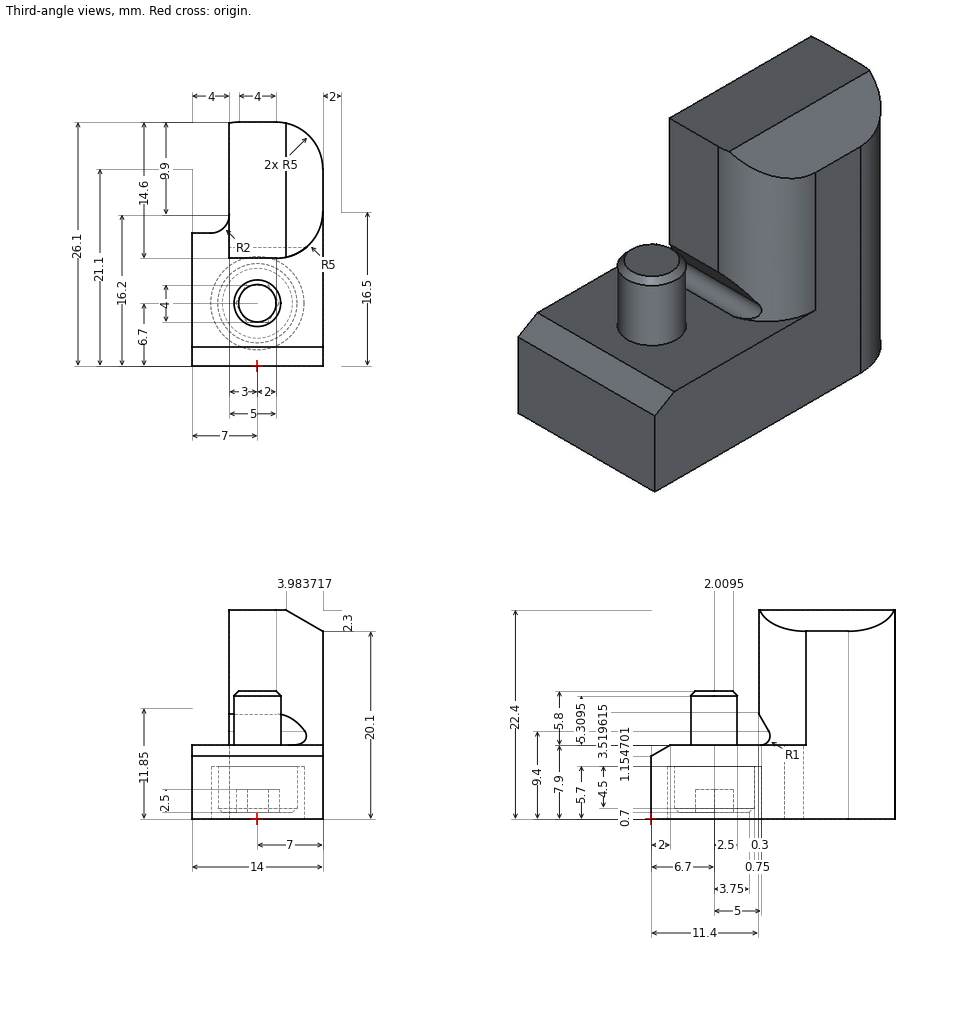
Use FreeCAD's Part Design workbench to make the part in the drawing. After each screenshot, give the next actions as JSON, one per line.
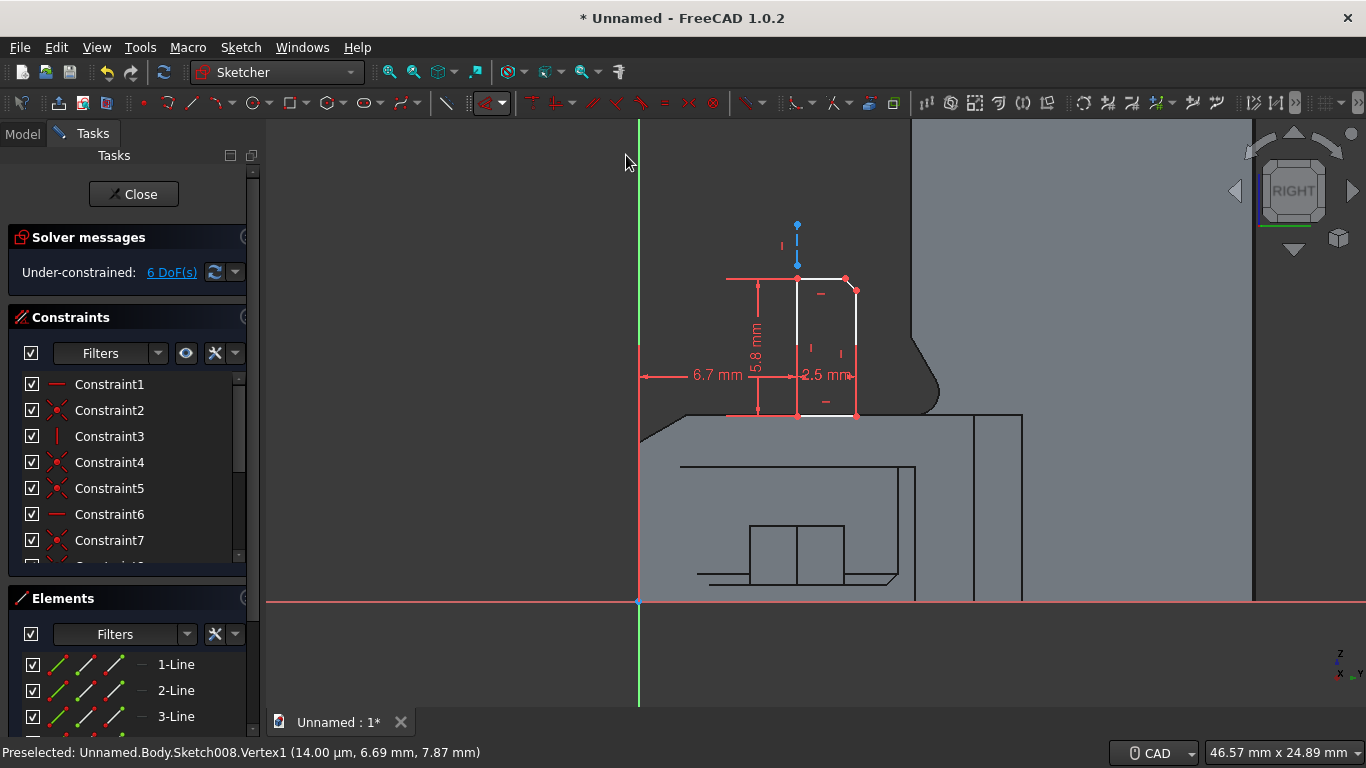
{"action": "left_click", "coordinate": [797, 416]}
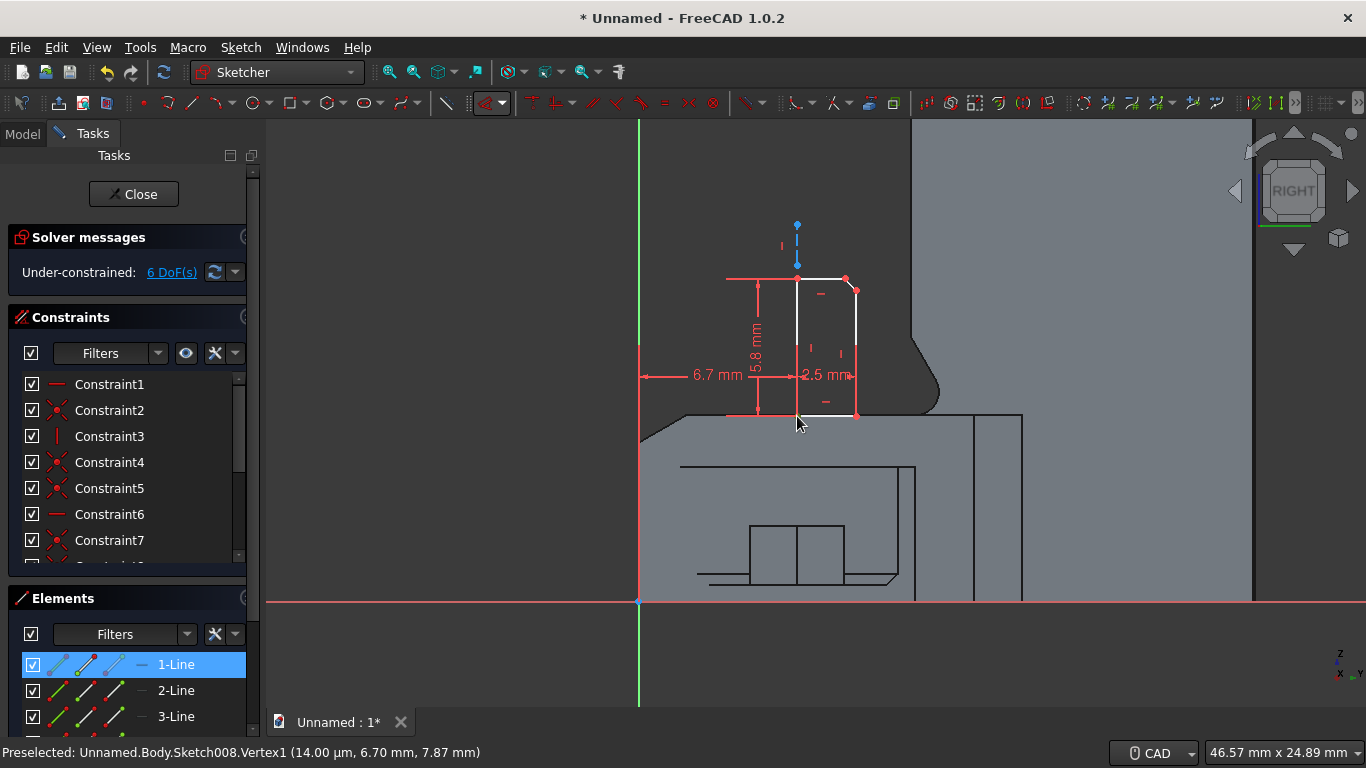
{"action": "key", "text": "i"}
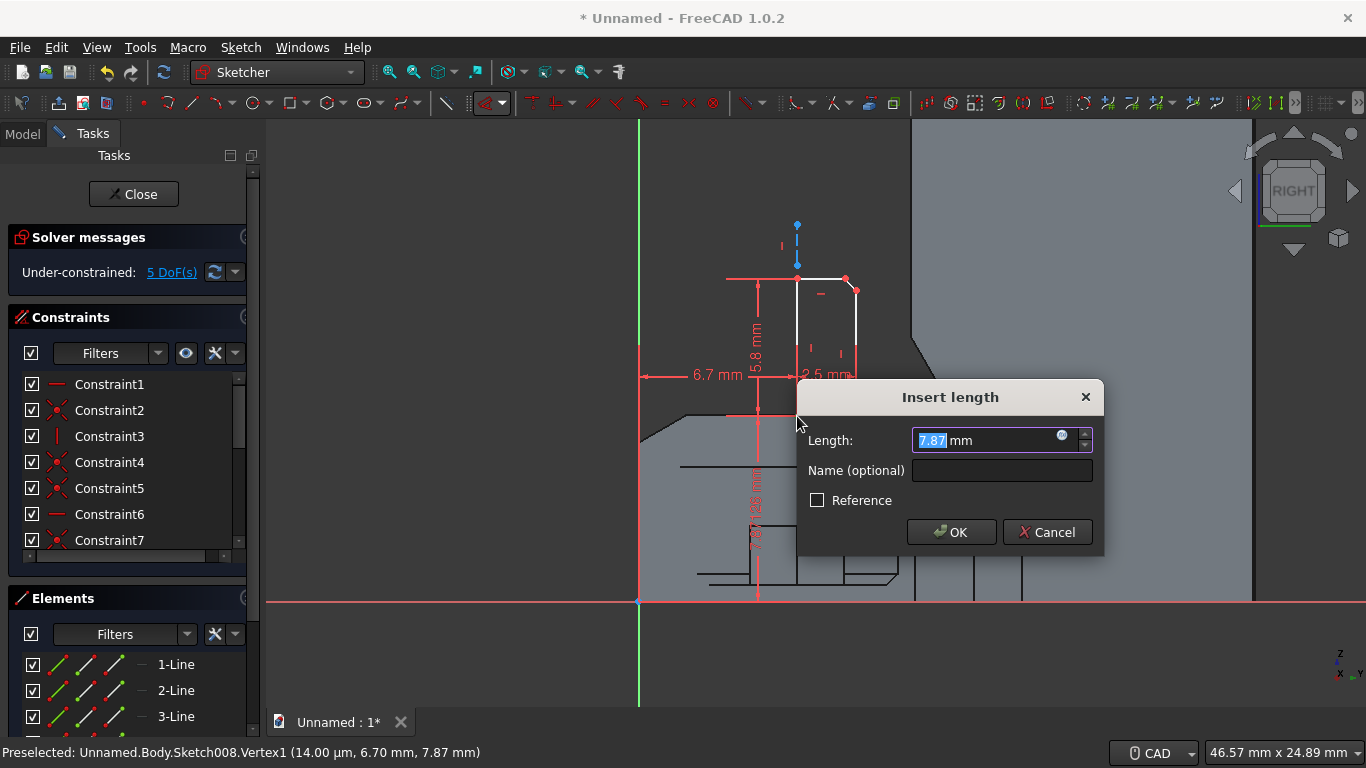
{"action": "type", "text": "7.9"}
{"action": "key", "text": "Return"}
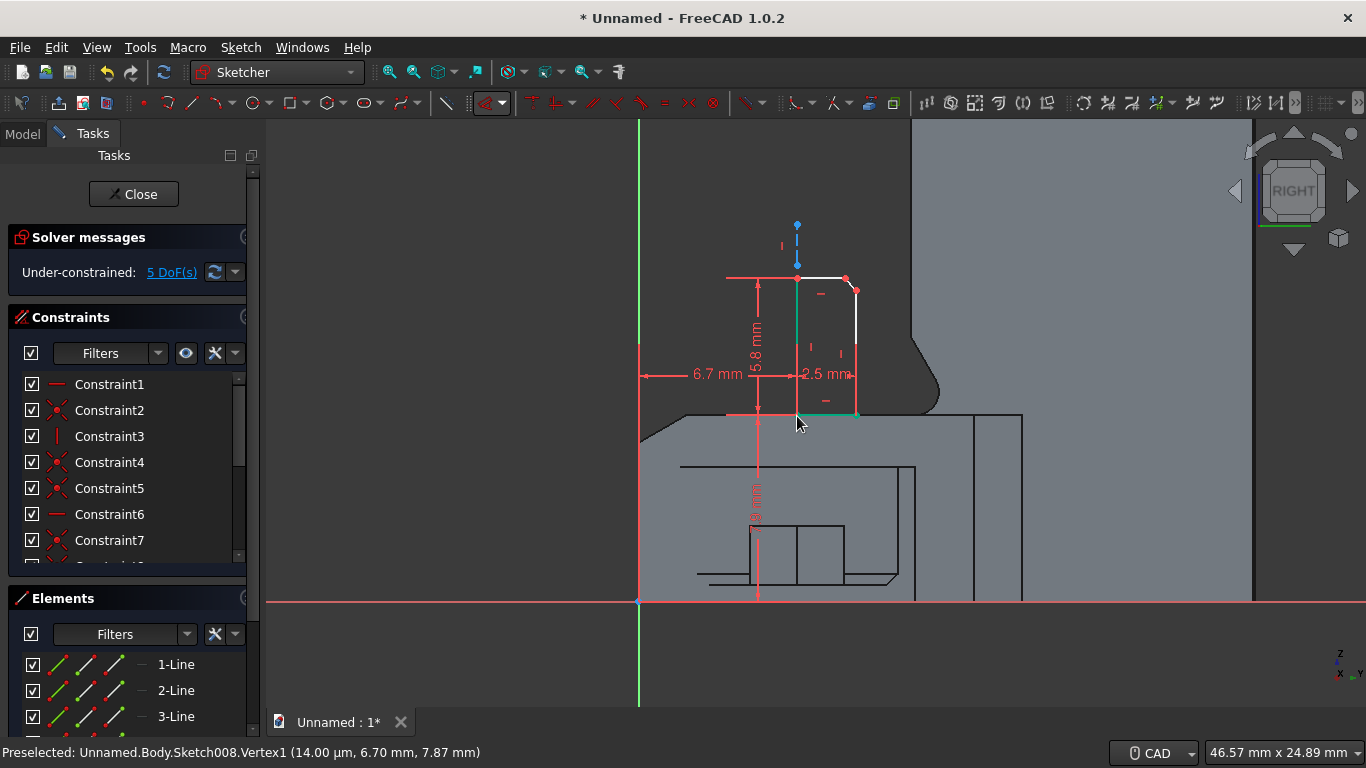
{"action": "left_click", "coordinate": [797, 266]}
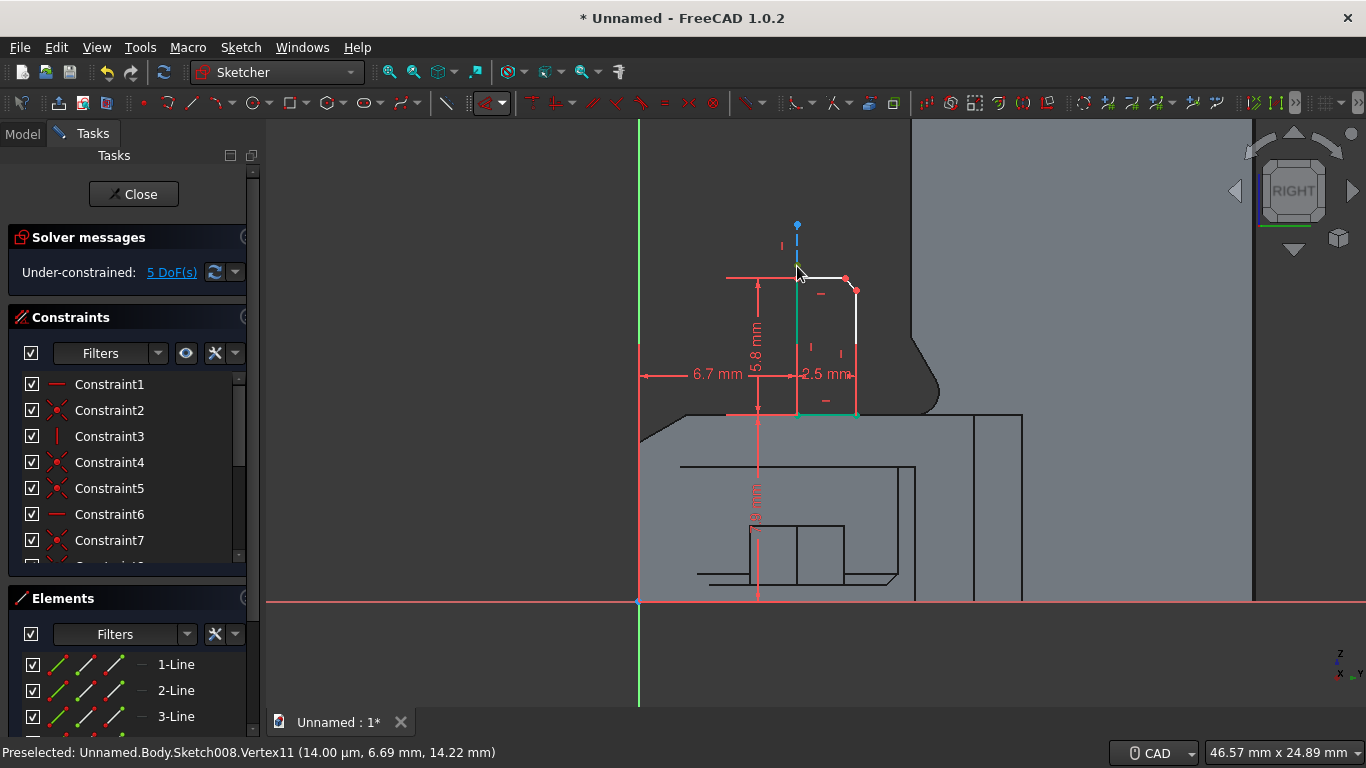
{"action": "left_click", "coordinate": [504, 104]}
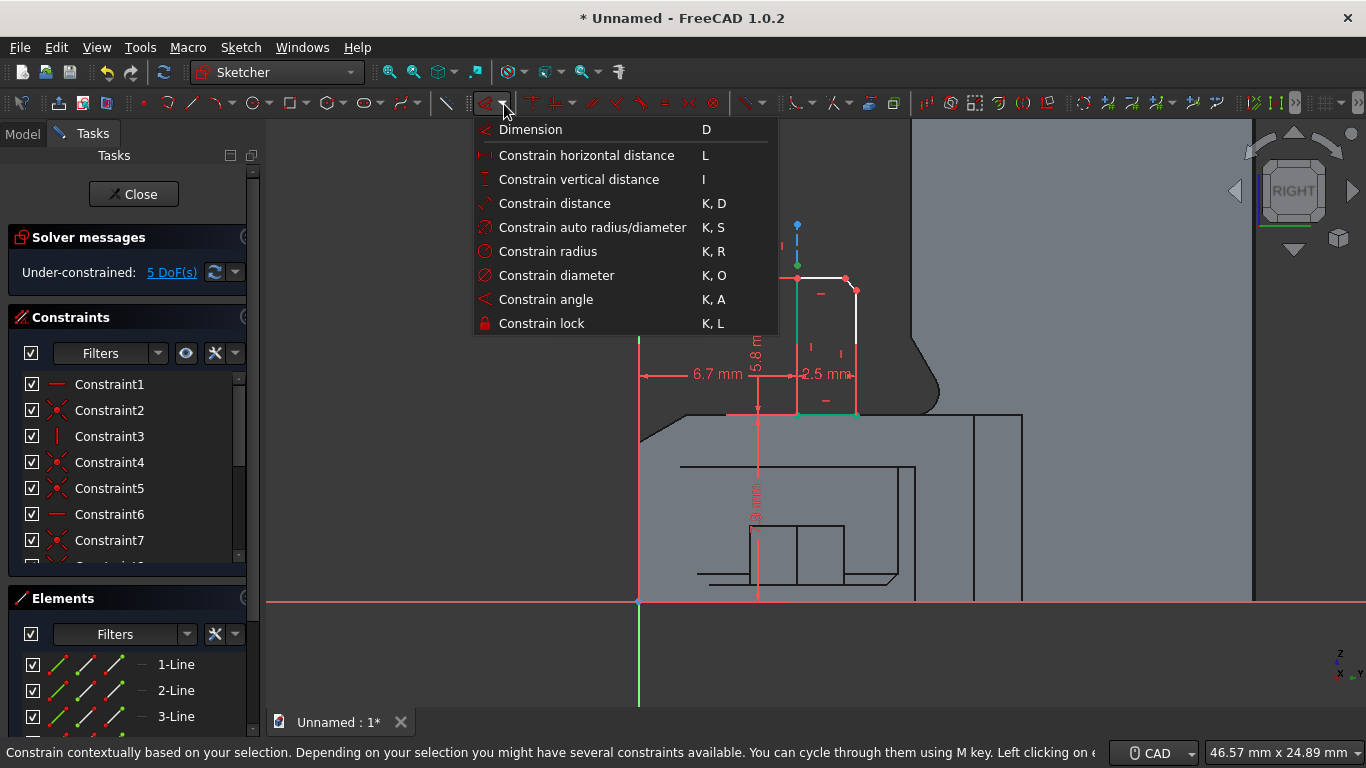
{"action": "left_click", "coordinate": [626, 155]}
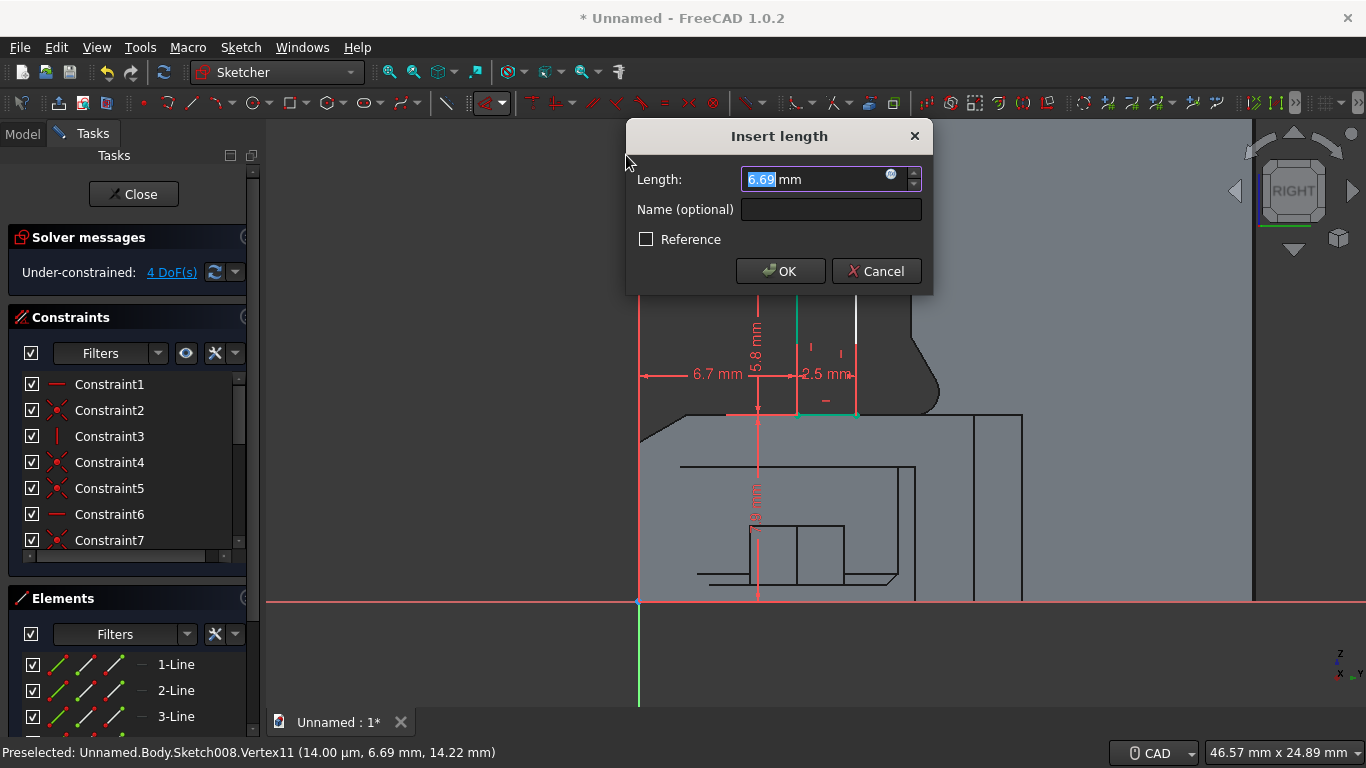
{"action": "type", "text": "6.7"}
{"action": "key", "text": "Return"}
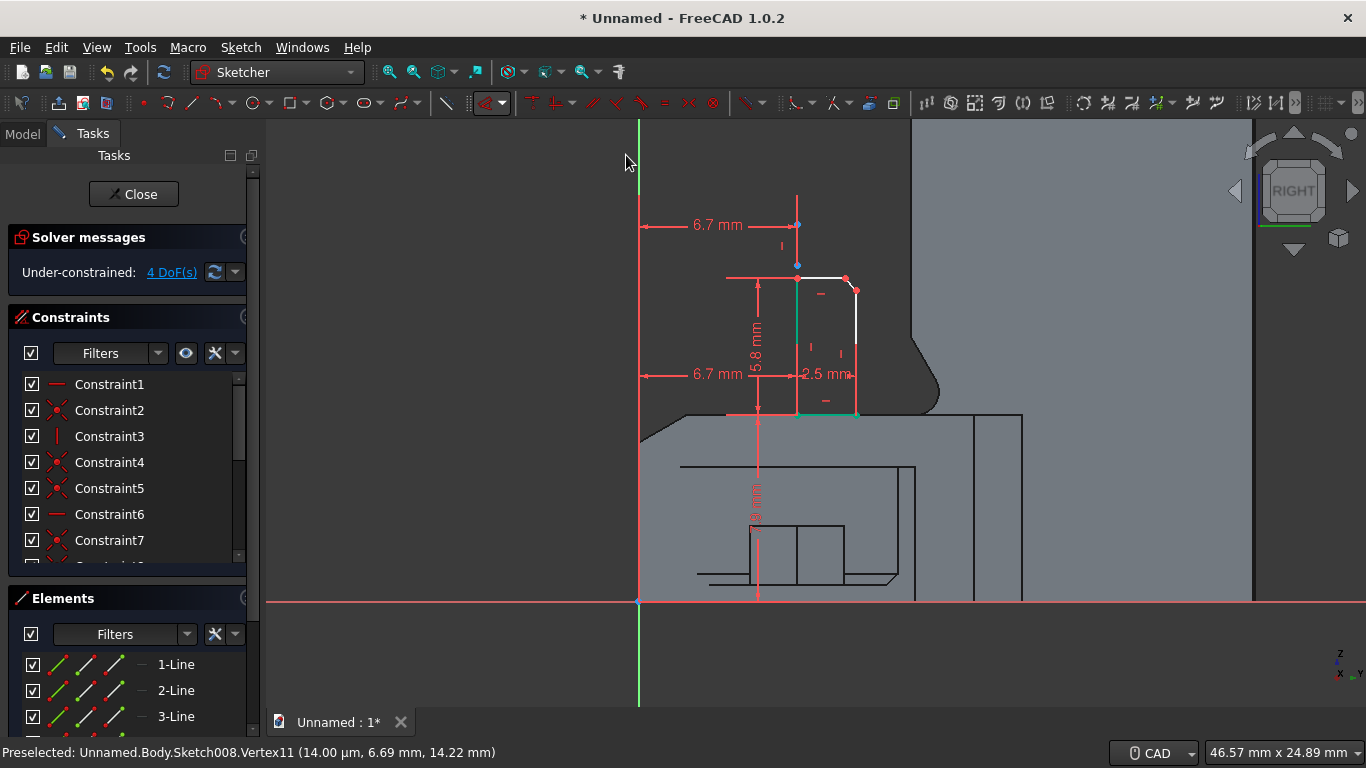
{"action": "left_click", "coordinate": [856, 378]}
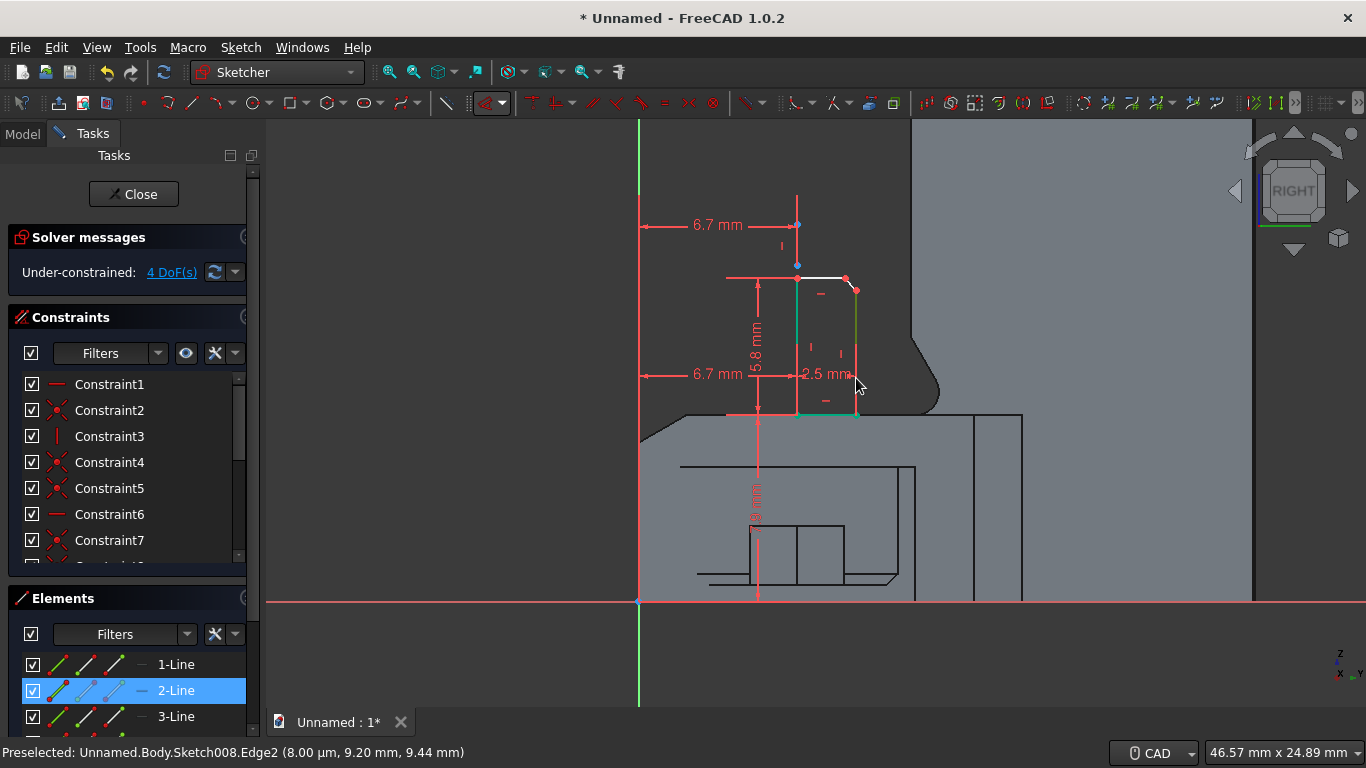
{"action": "left_click", "coordinate": [504, 104]}